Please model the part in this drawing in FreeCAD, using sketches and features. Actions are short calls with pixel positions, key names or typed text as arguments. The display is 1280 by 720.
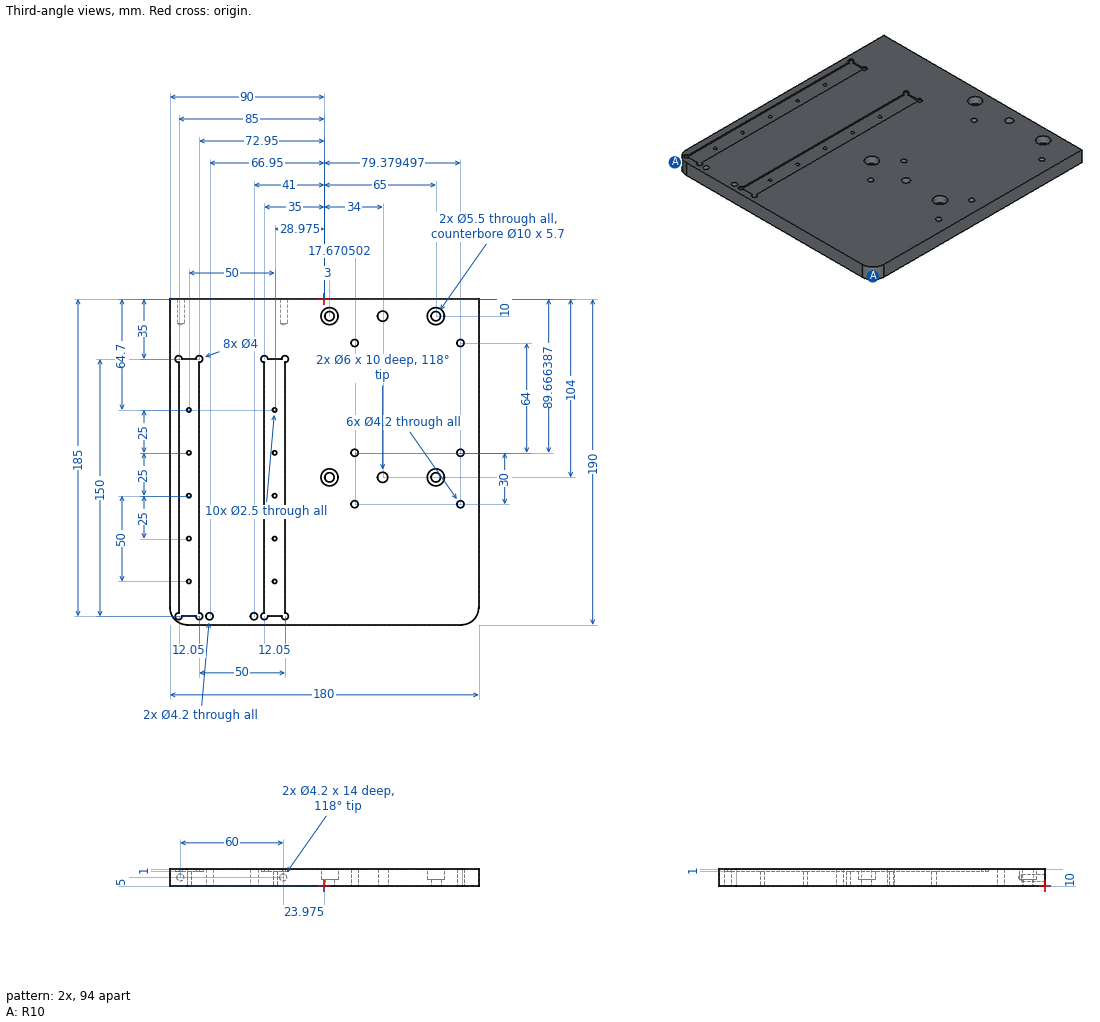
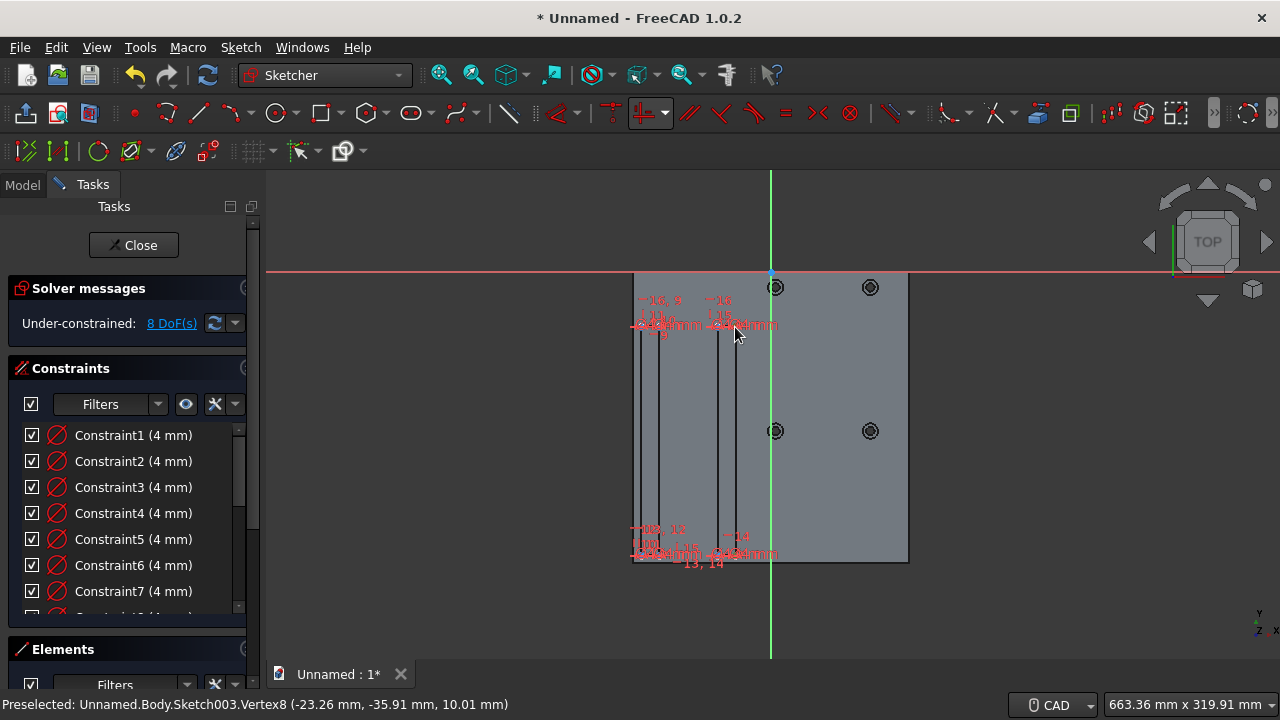
click(668, 114)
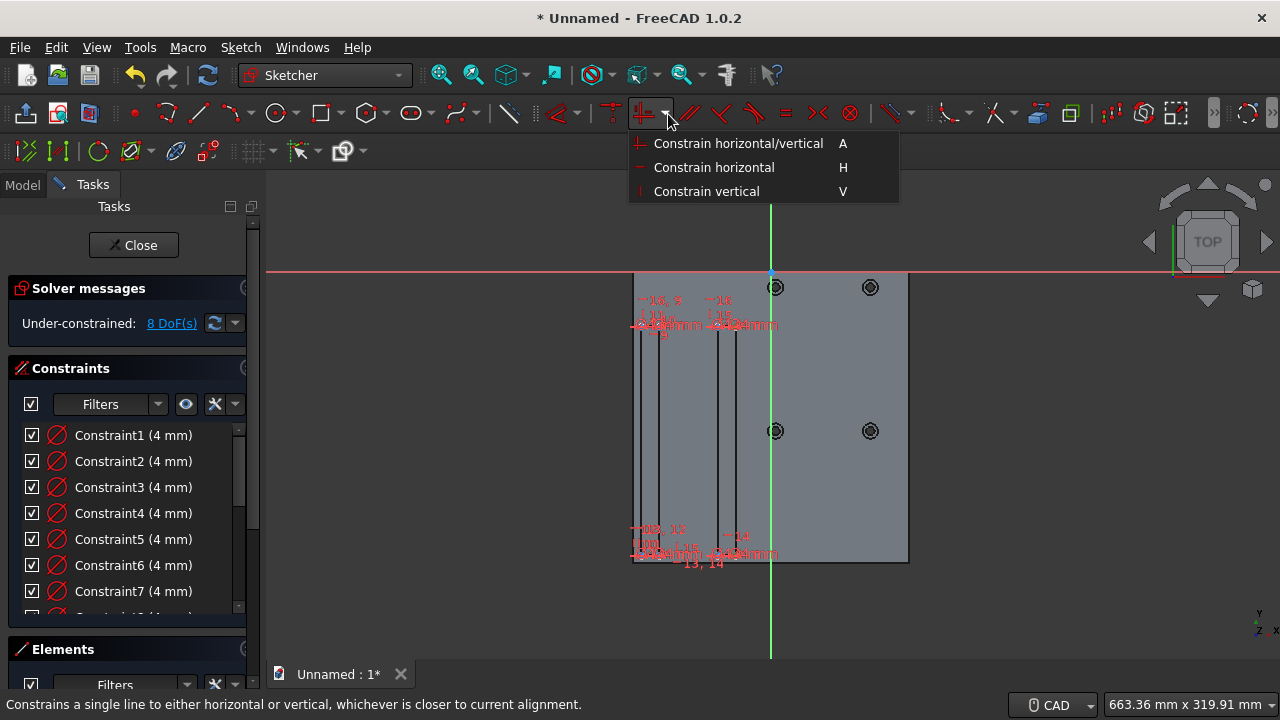
click(764, 191)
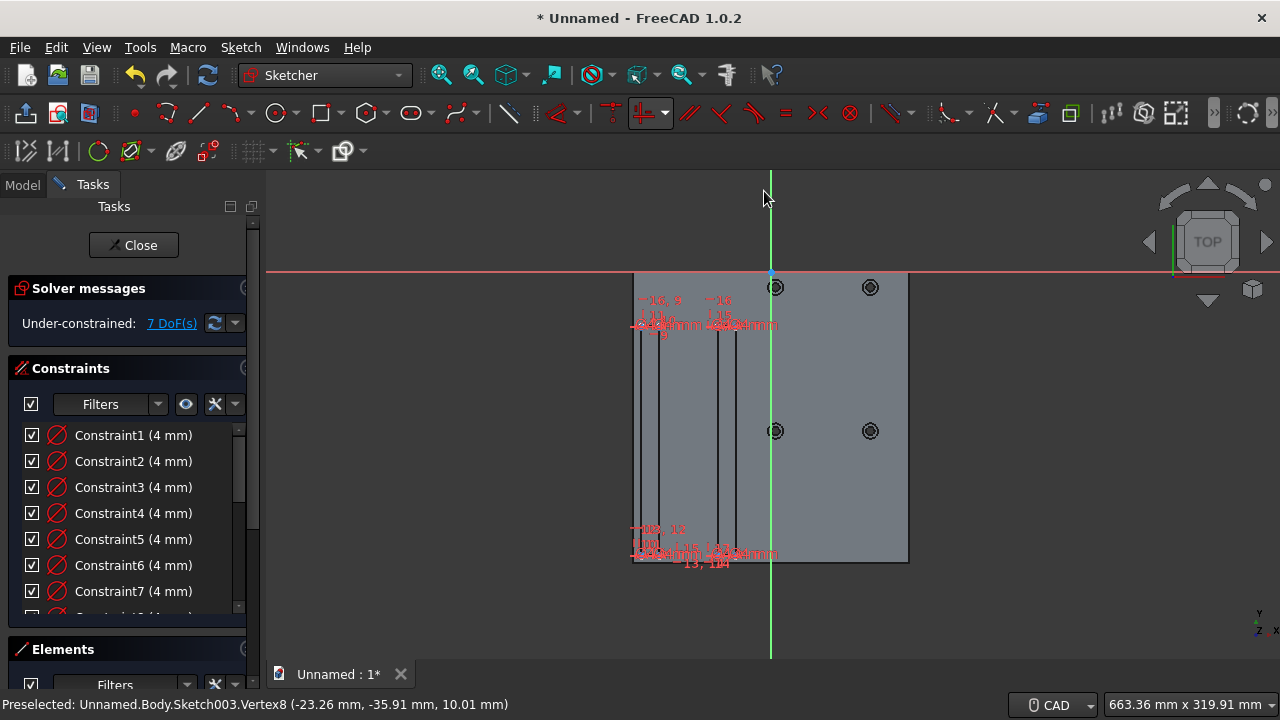
scroll(717, 327, up, 4)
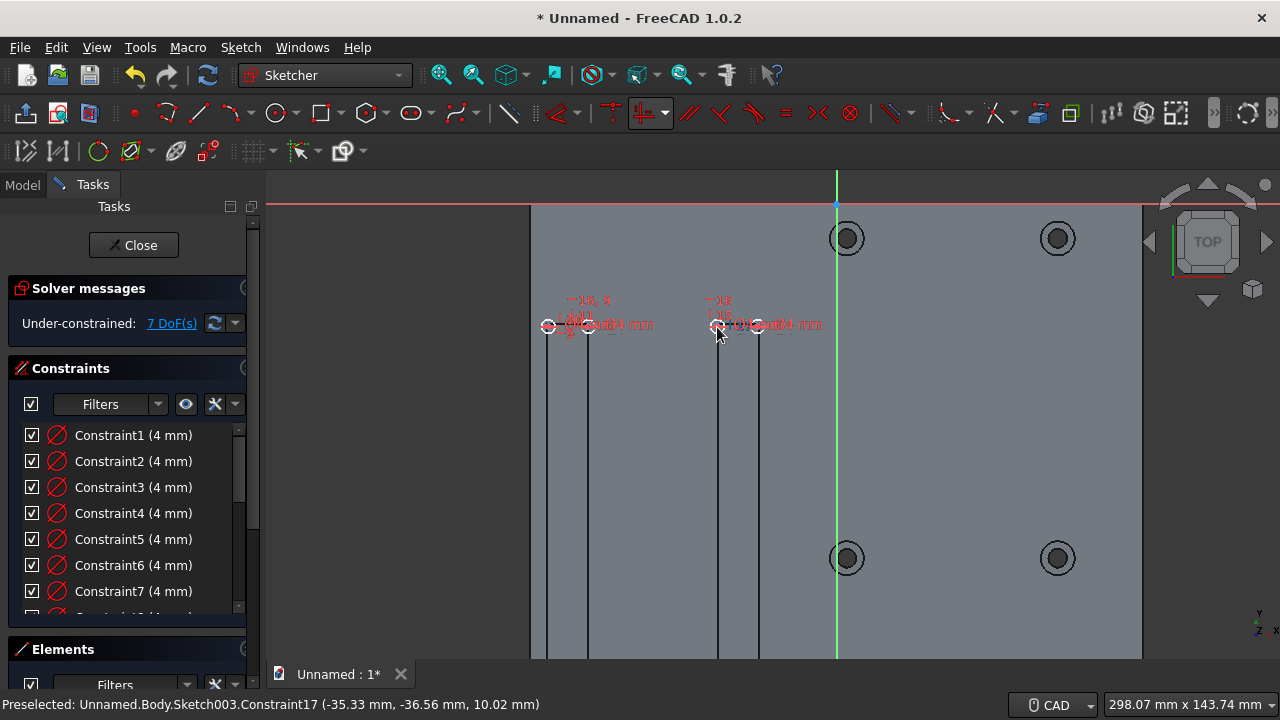
click(717, 327)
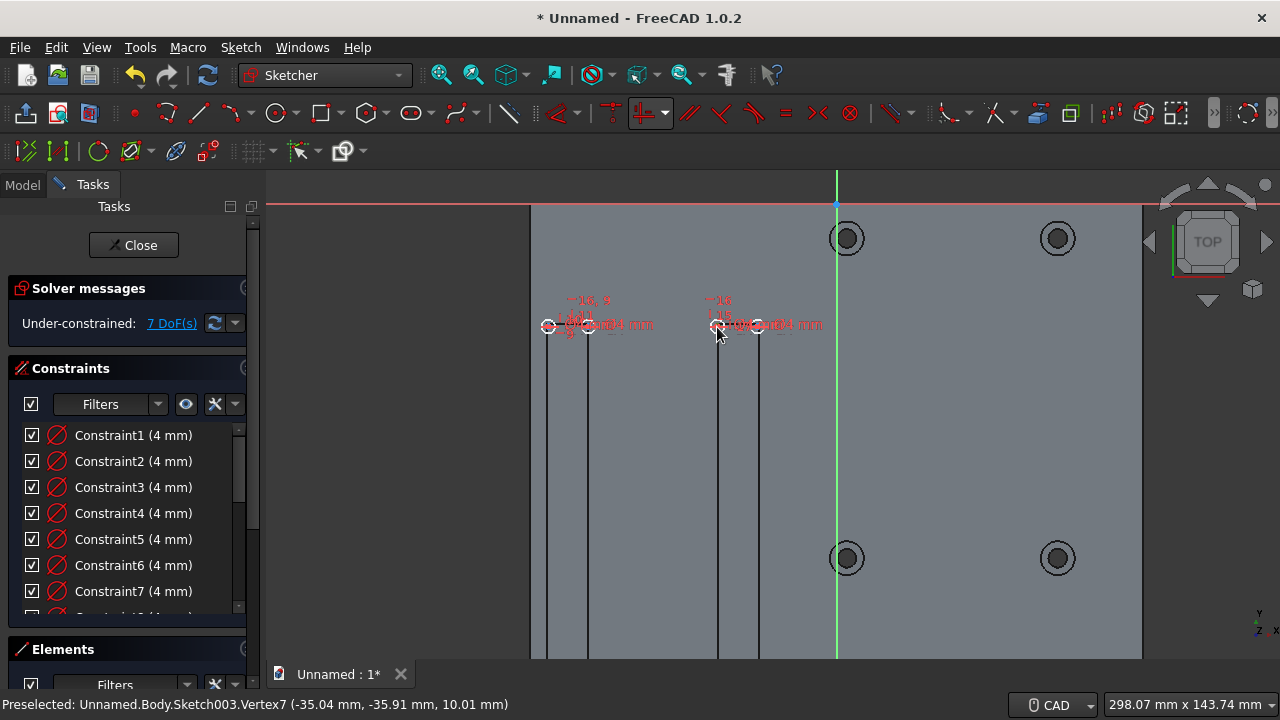
click(758, 327)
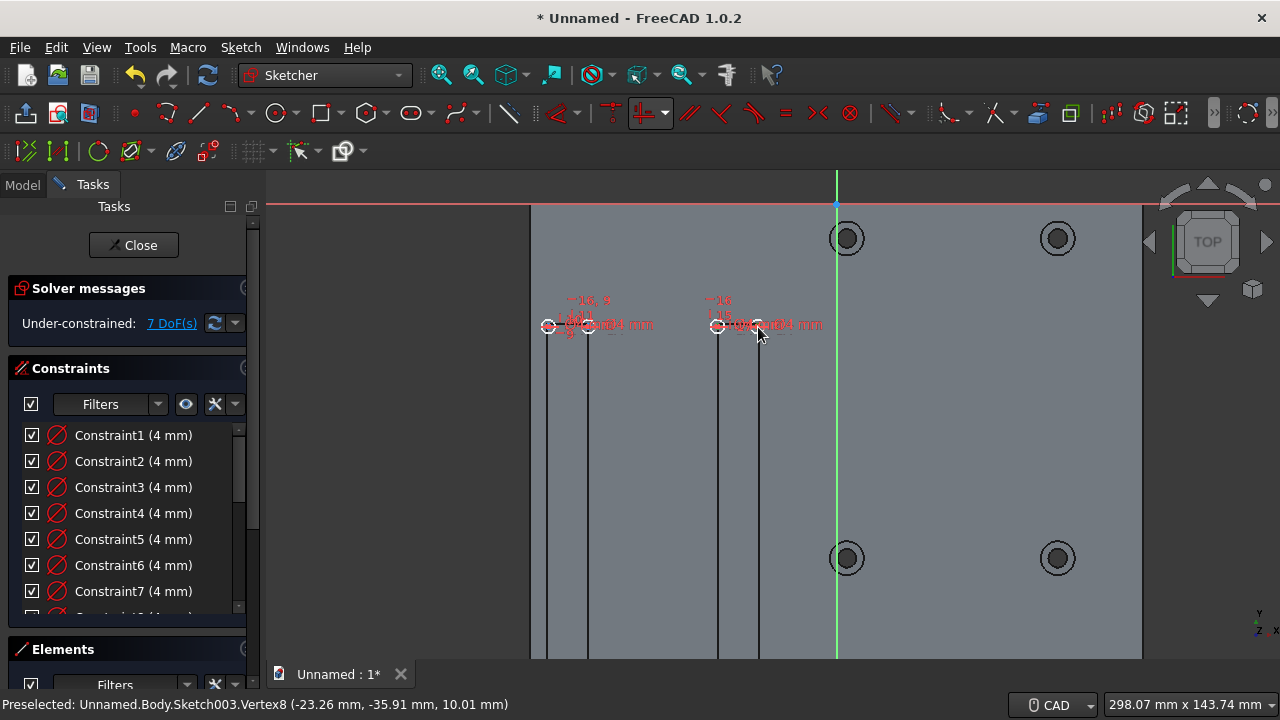
click(668, 114)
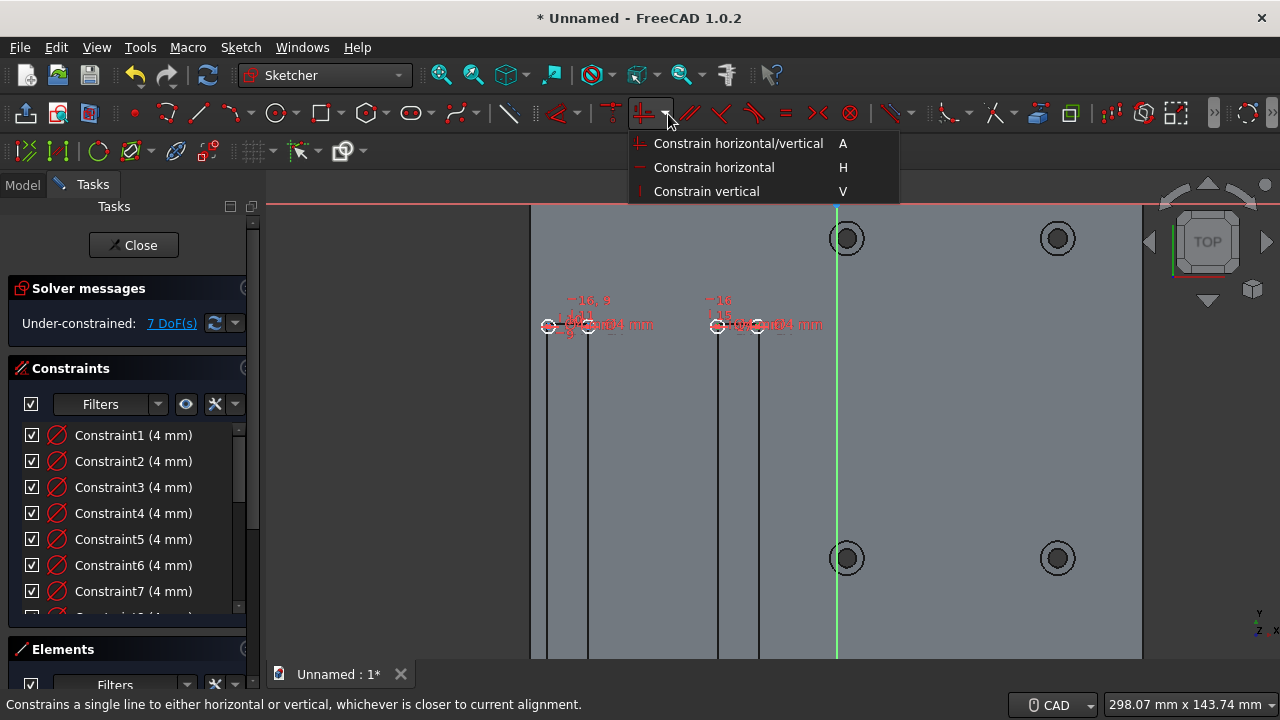
click(764, 167)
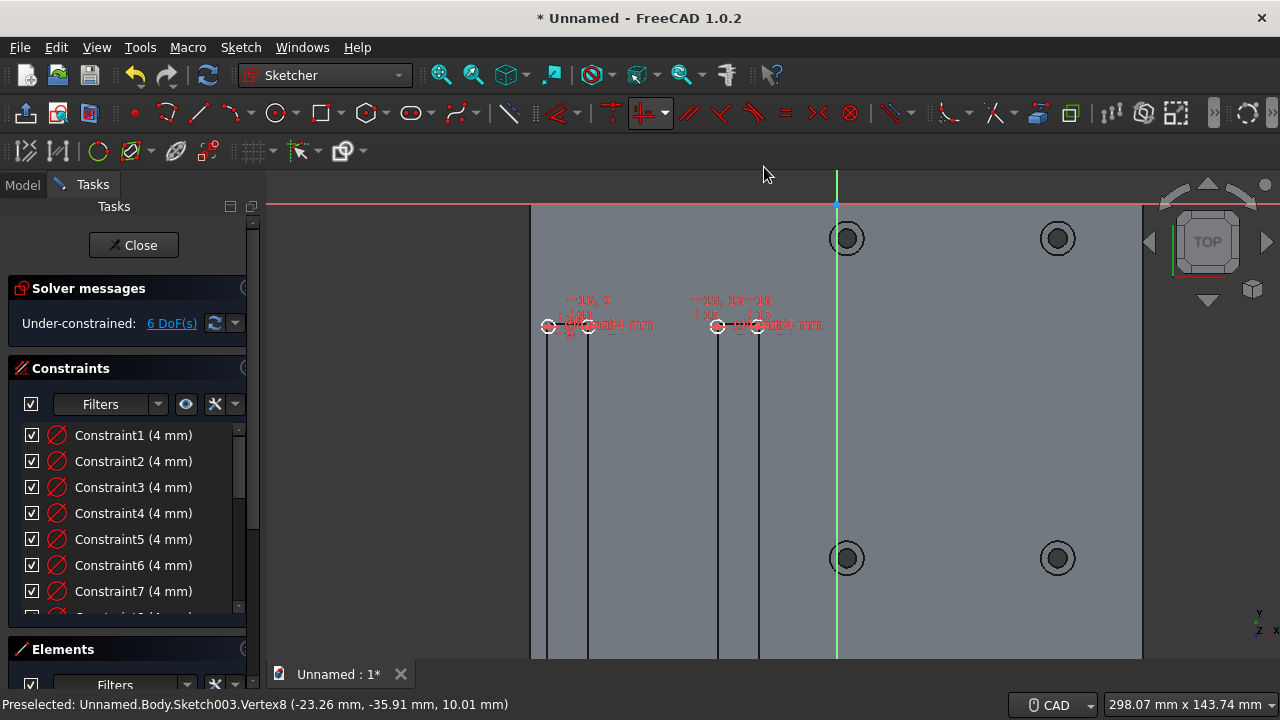
click(588, 327)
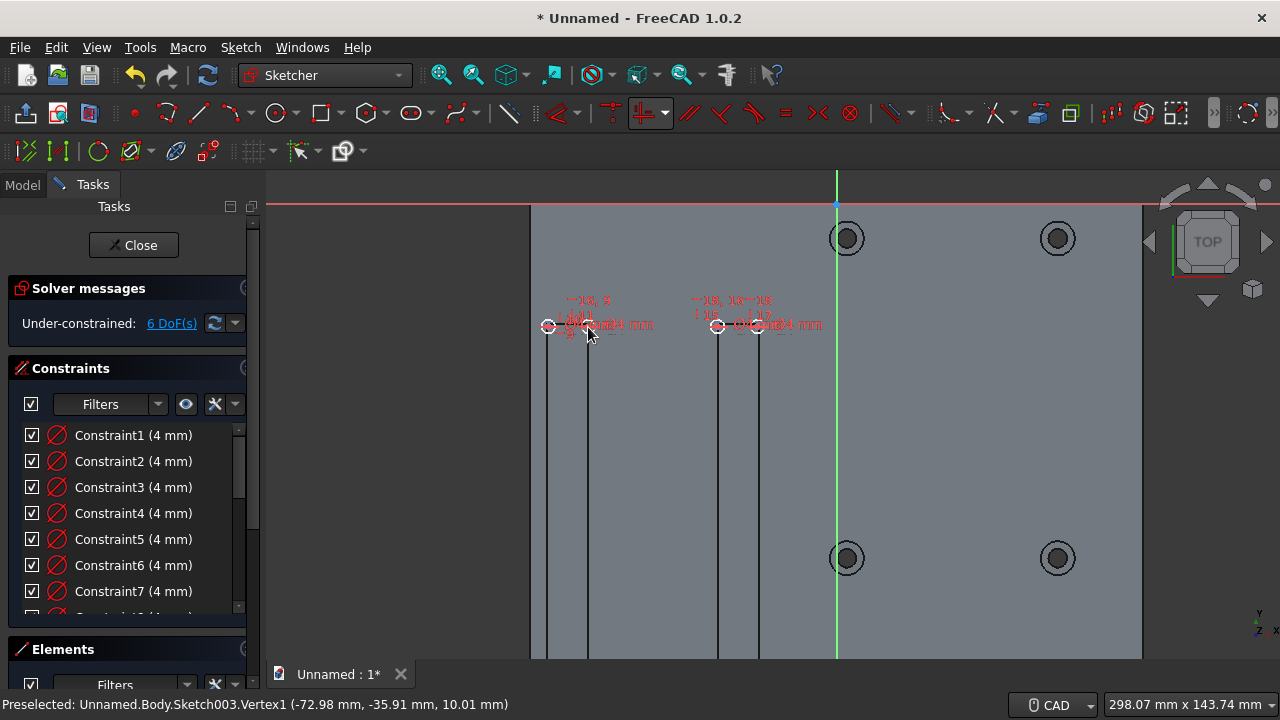
key(i)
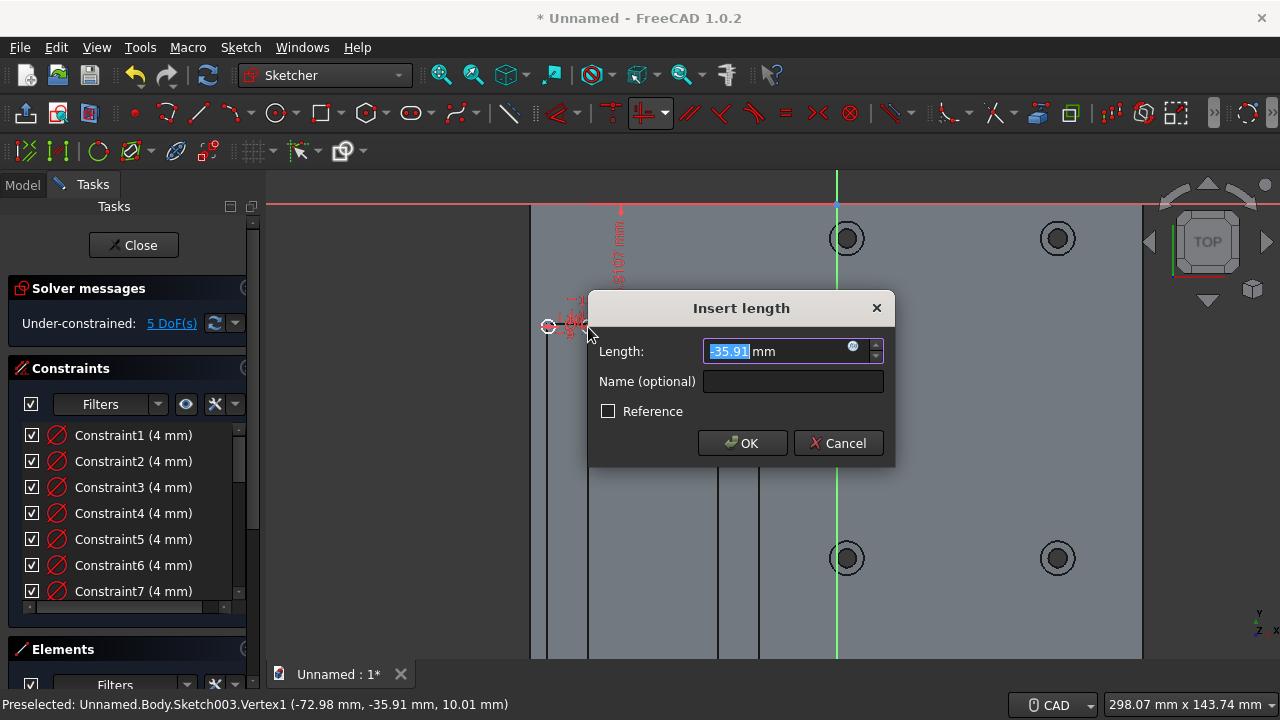
text(-35)
key(Return)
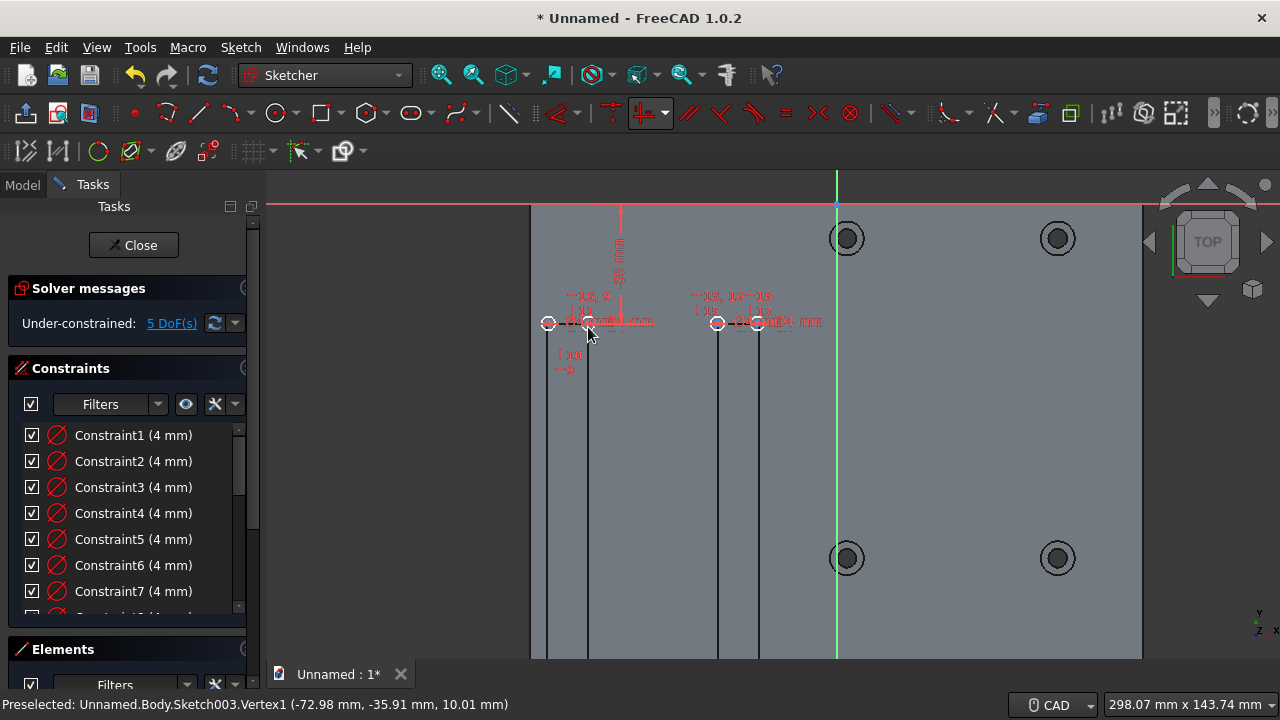
click(548, 324)